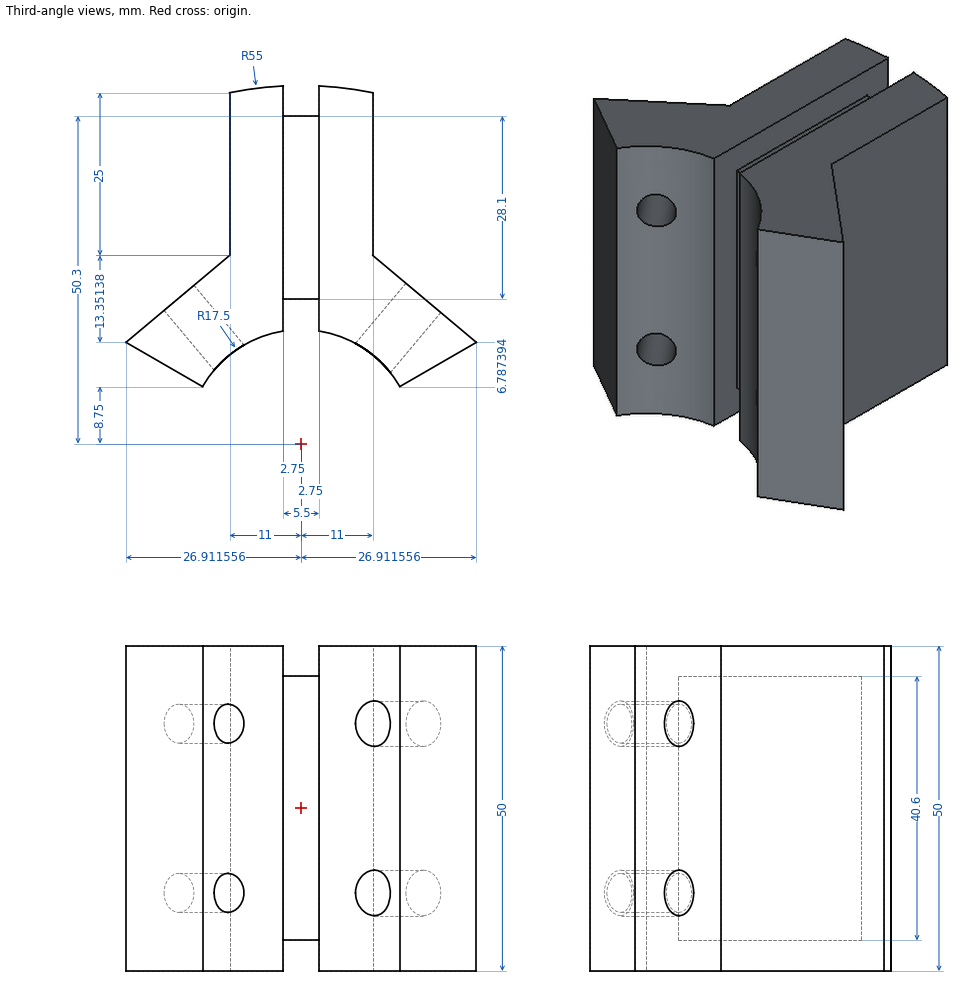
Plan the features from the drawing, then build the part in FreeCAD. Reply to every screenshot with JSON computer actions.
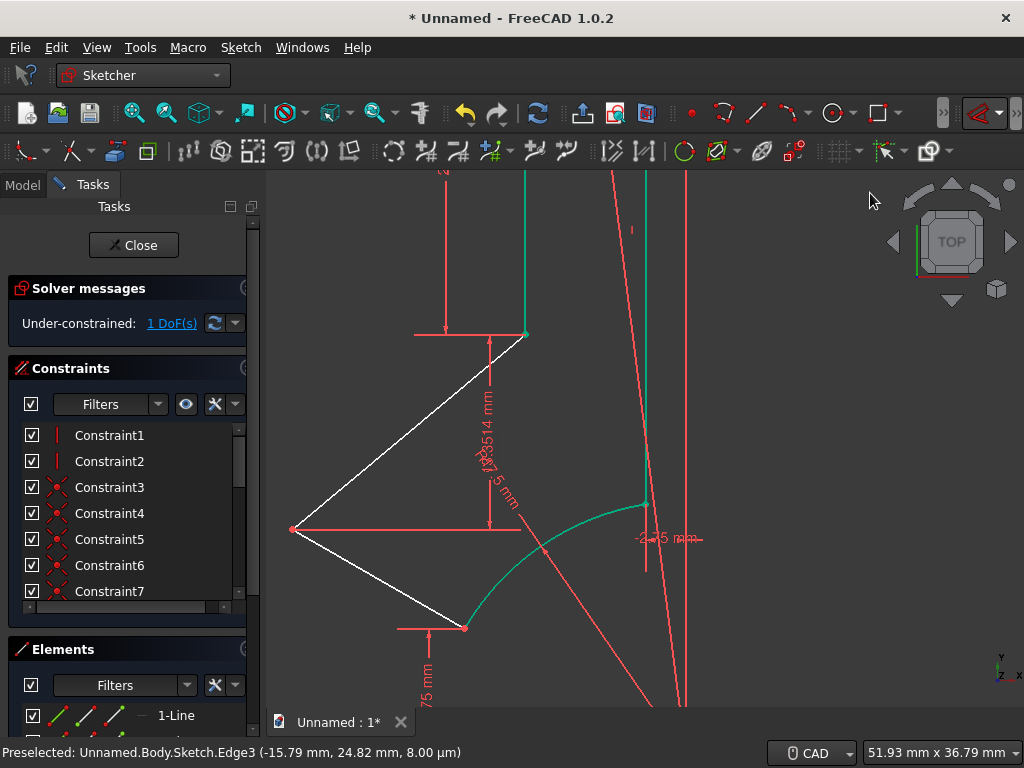
{"action": "scroll", "coordinate": [647, 506], "scroll_direction": "down", "scroll_amount": 4}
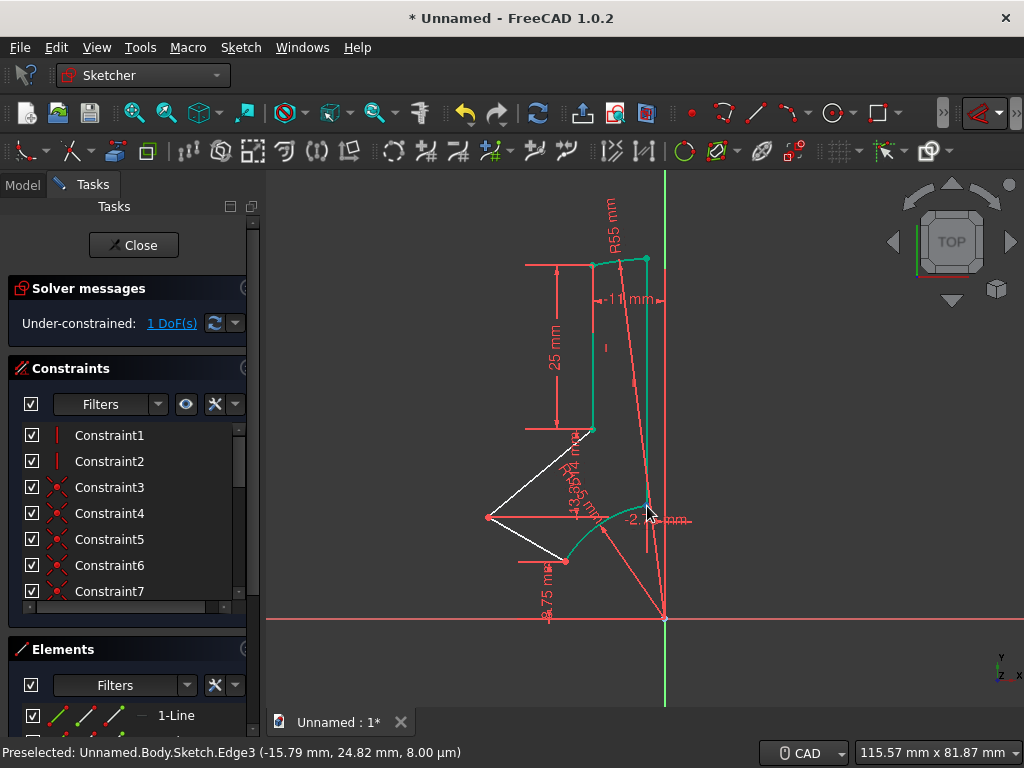
{"action": "left_click", "coordinate": [488, 517]}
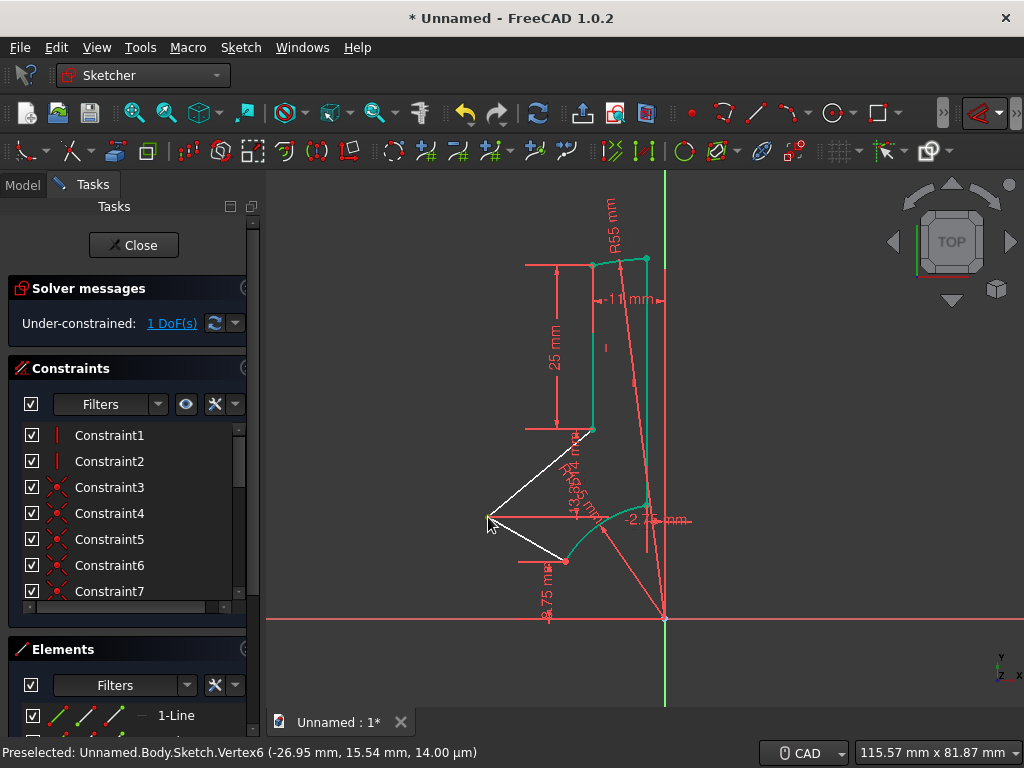
{"action": "left_click", "coordinate": [1002, 114]}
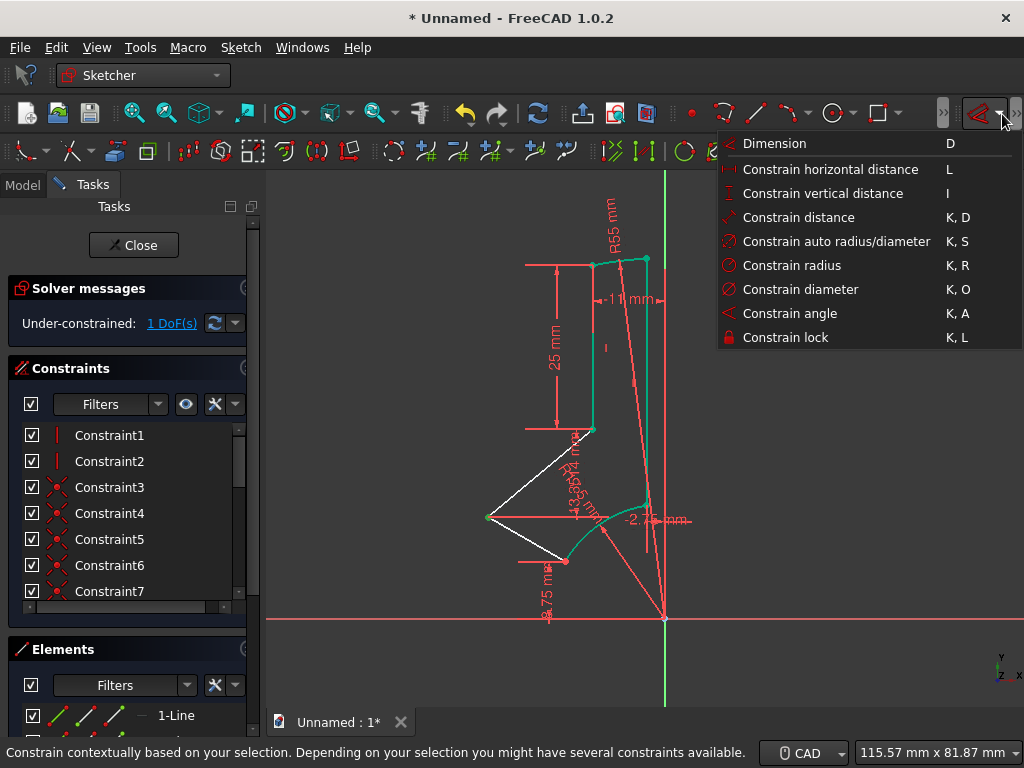
{"action": "left_click", "coordinate": [870, 169]}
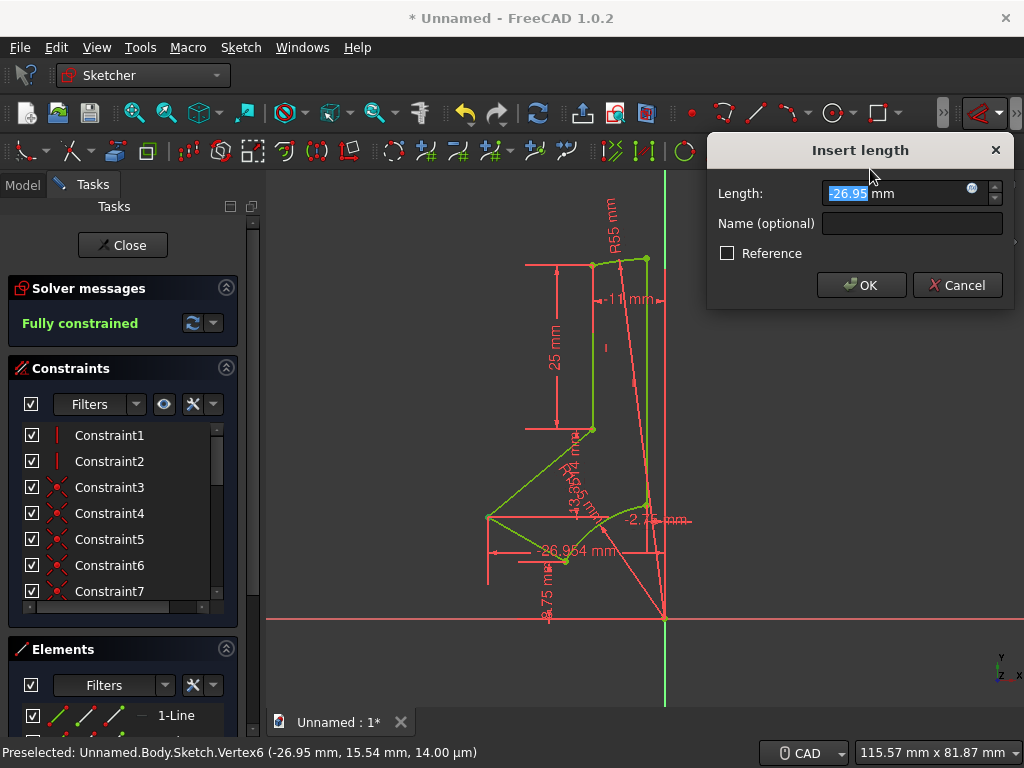
{"action": "type", "text": "-26.911556"}
{"action": "key", "text": "Return"}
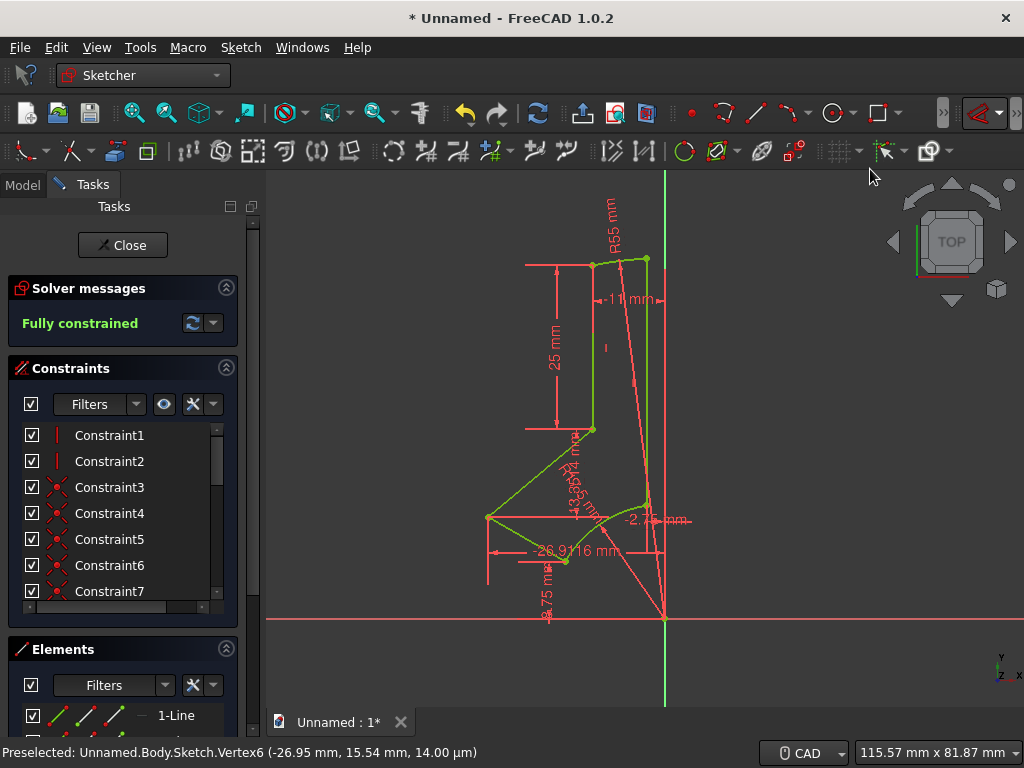
{"action": "left_click", "coordinate": [123, 245]}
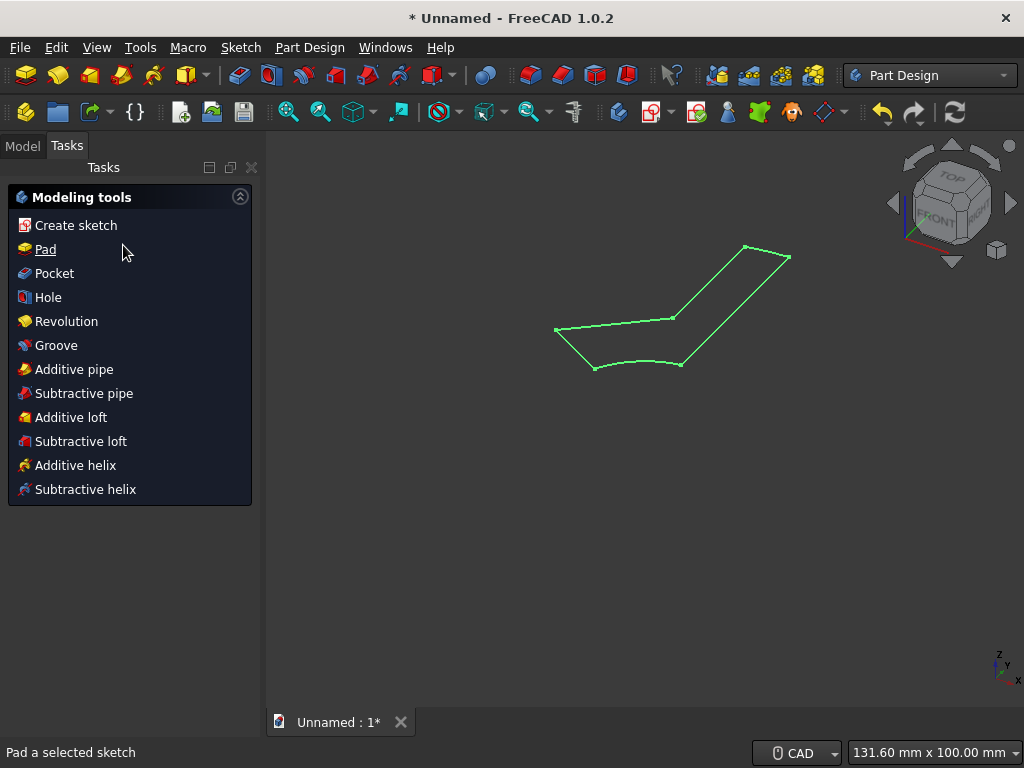
{"action": "left_click", "coordinate": [26, 76]}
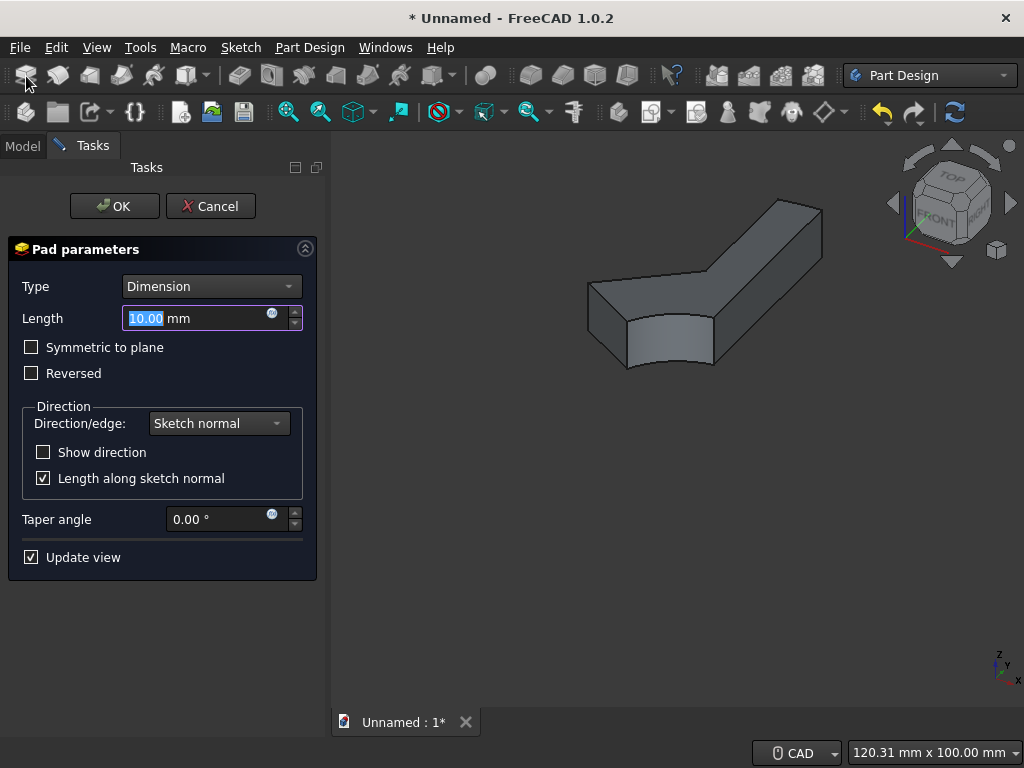
{"action": "type", "text": "50"}
{"action": "key", "text": "Tab"}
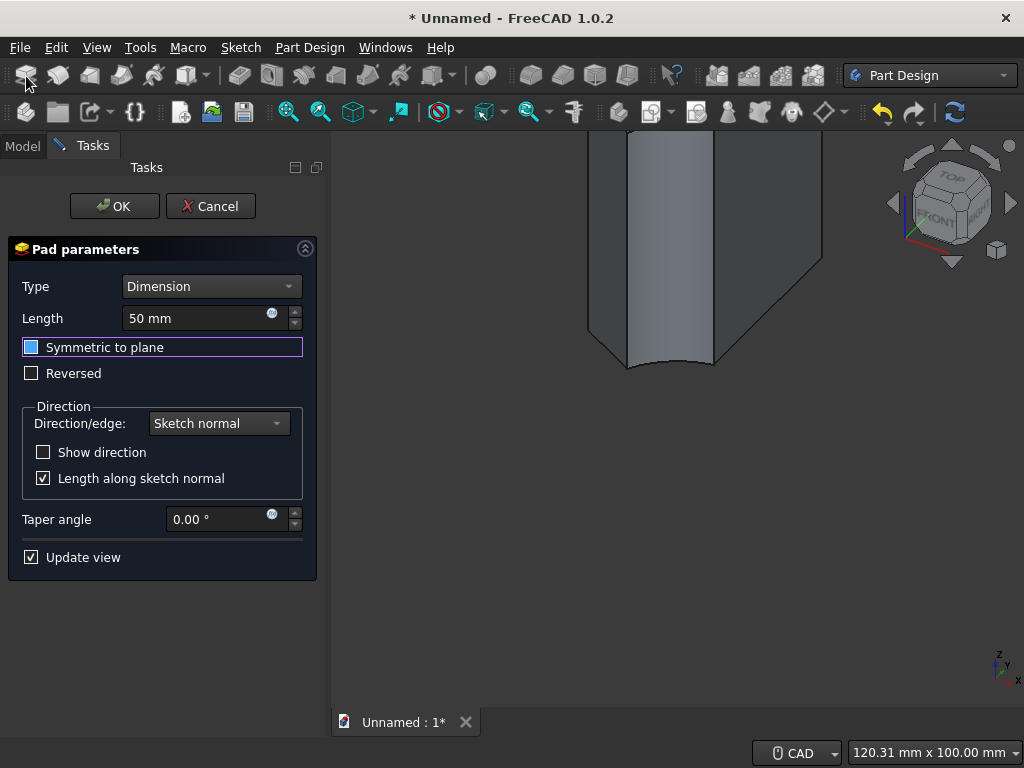
{"action": "left_click", "coordinate": [30, 347]}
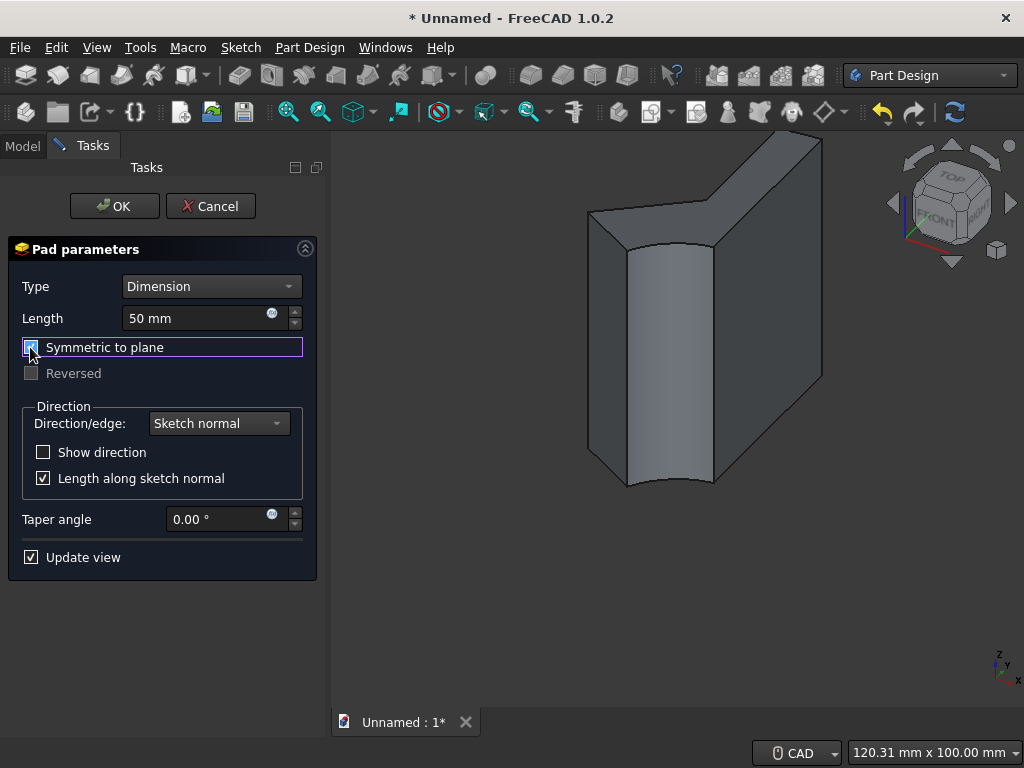
{"action": "left_click", "coordinate": [115, 206]}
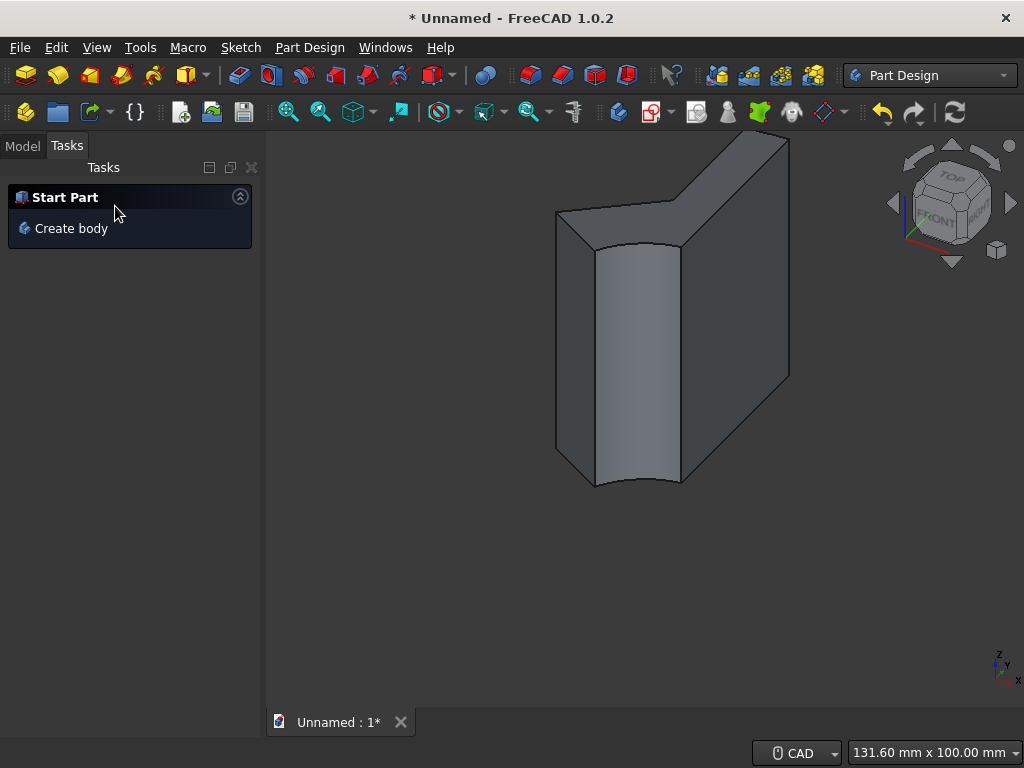
{"action": "left_click", "coordinate": [290, 112]}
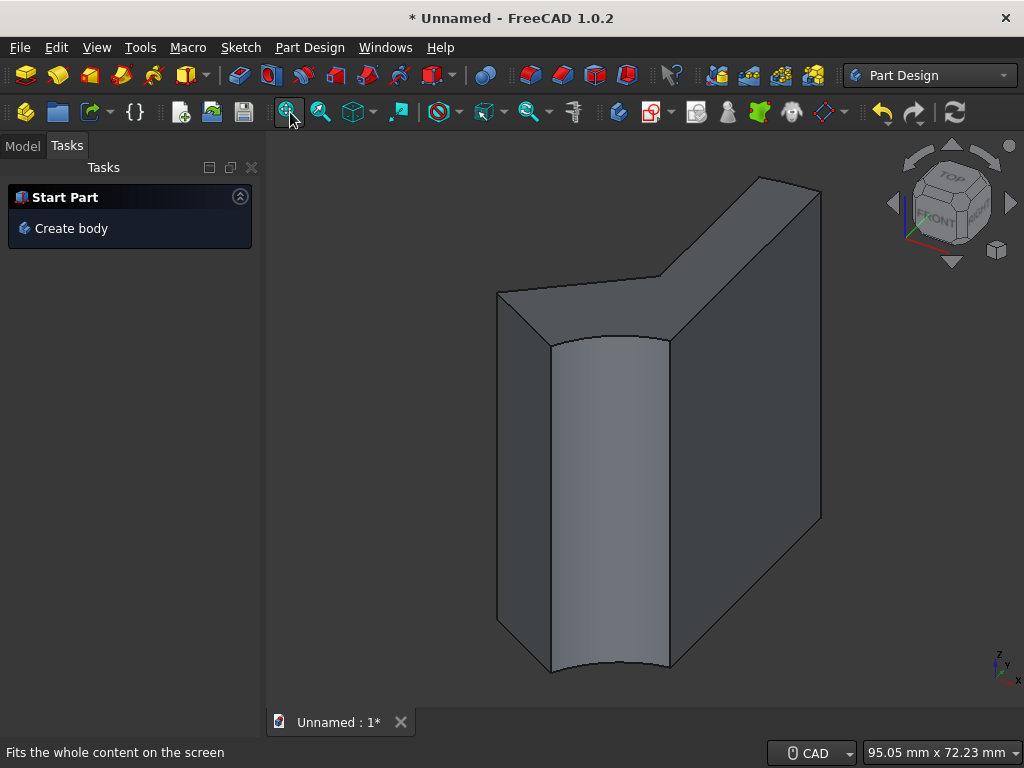
{"action": "left_click", "coordinate": [620, 112]}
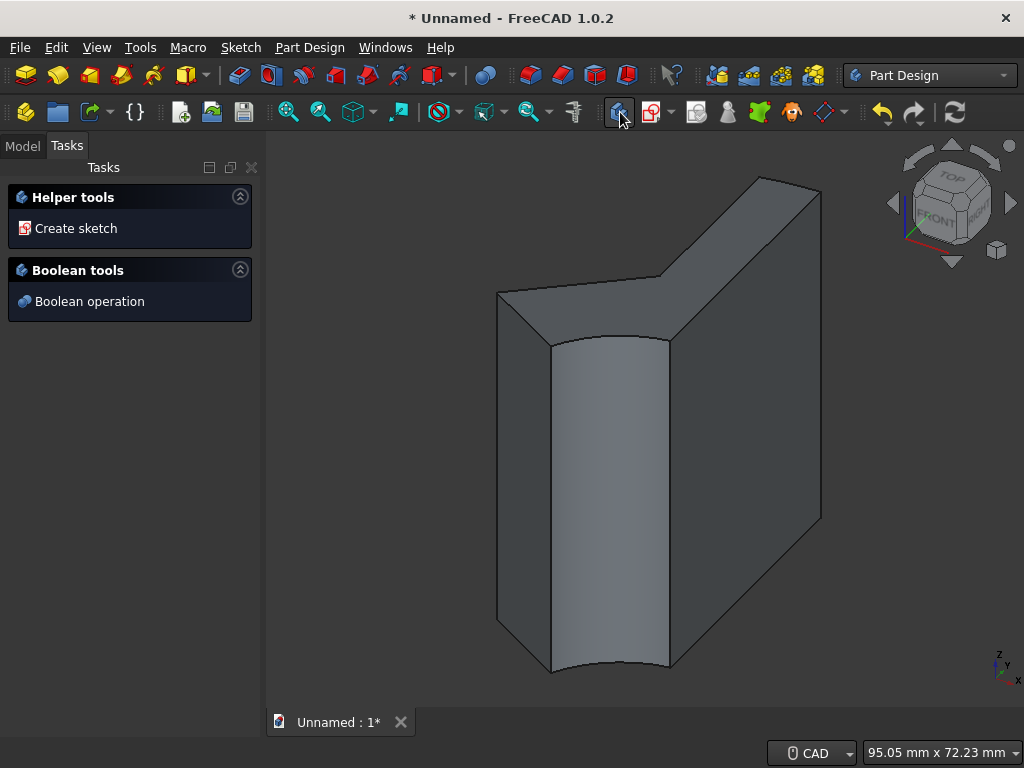
{"action": "left_click", "coordinate": [306, 667]}